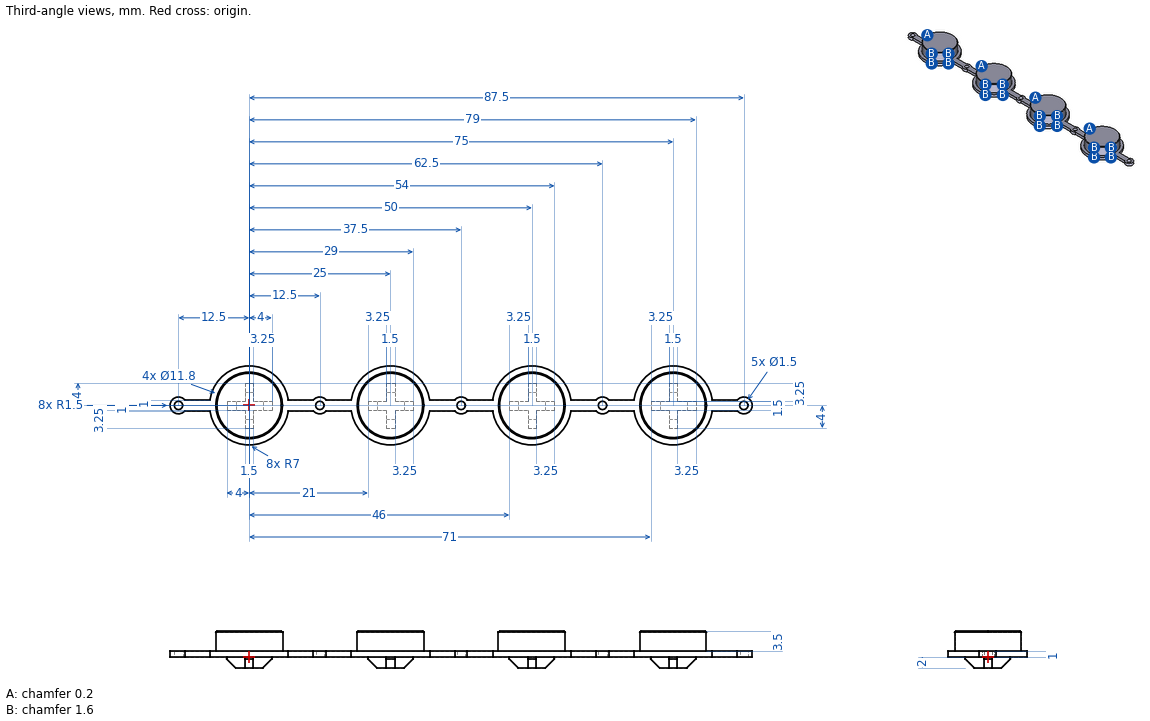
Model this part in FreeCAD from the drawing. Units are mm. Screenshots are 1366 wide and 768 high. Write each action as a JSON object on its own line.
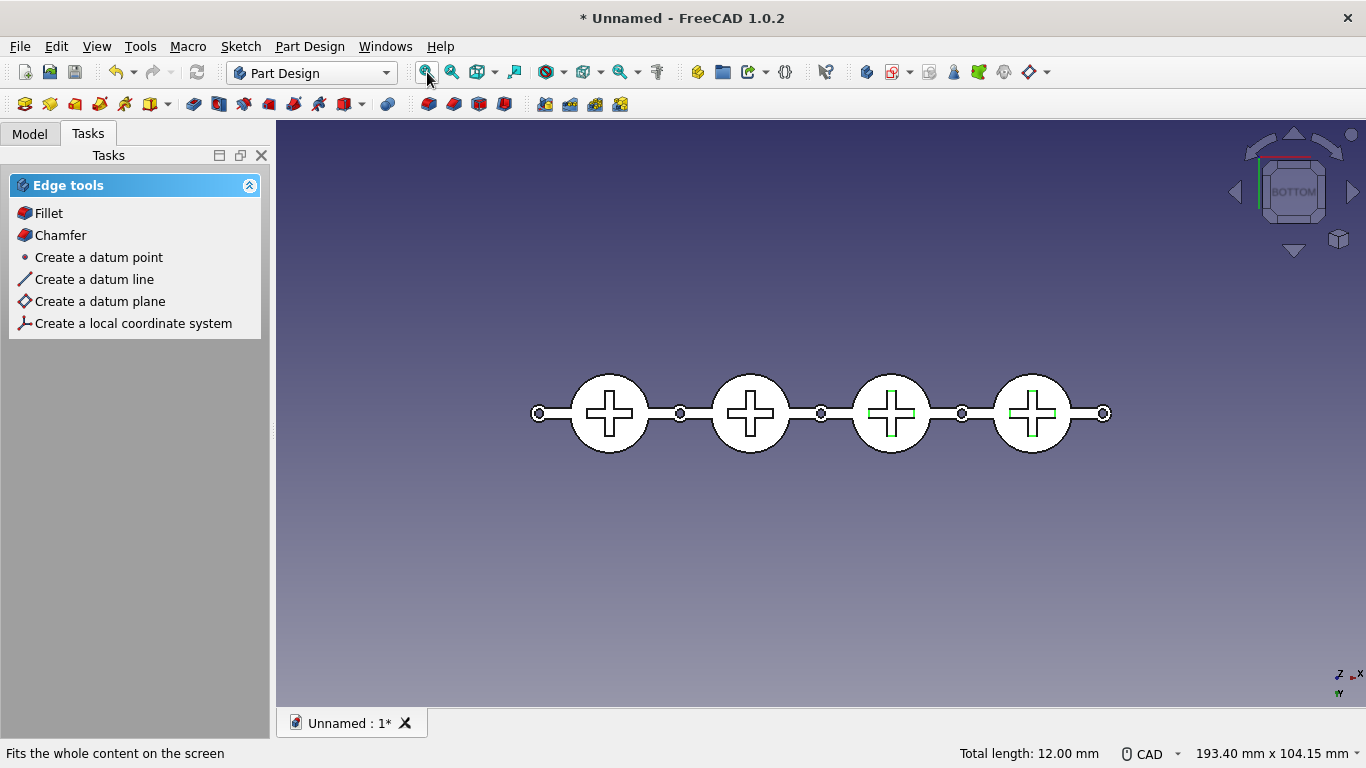
{"action": "key", "text": "4"}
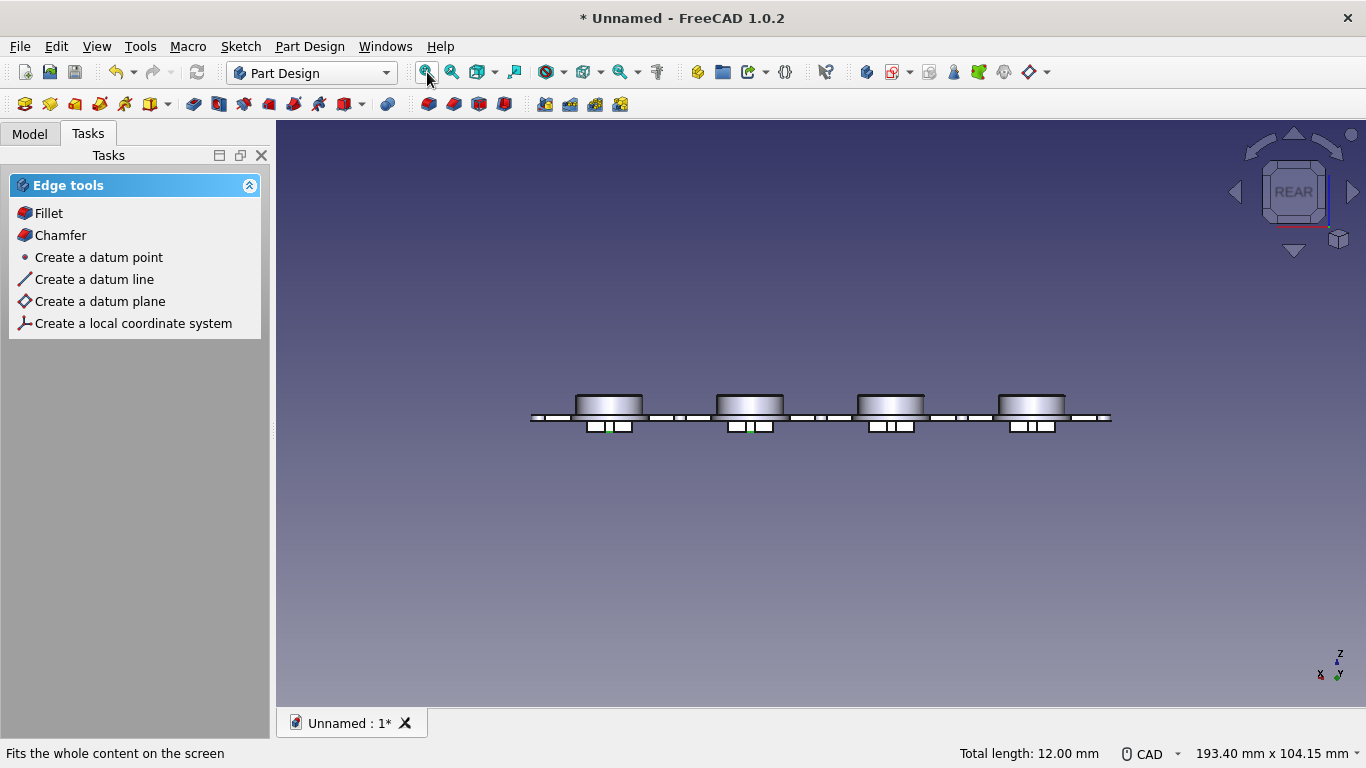
{"action": "scroll", "coordinate": [914, 431], "scroll_direction": "up", "scroll_amount": 8}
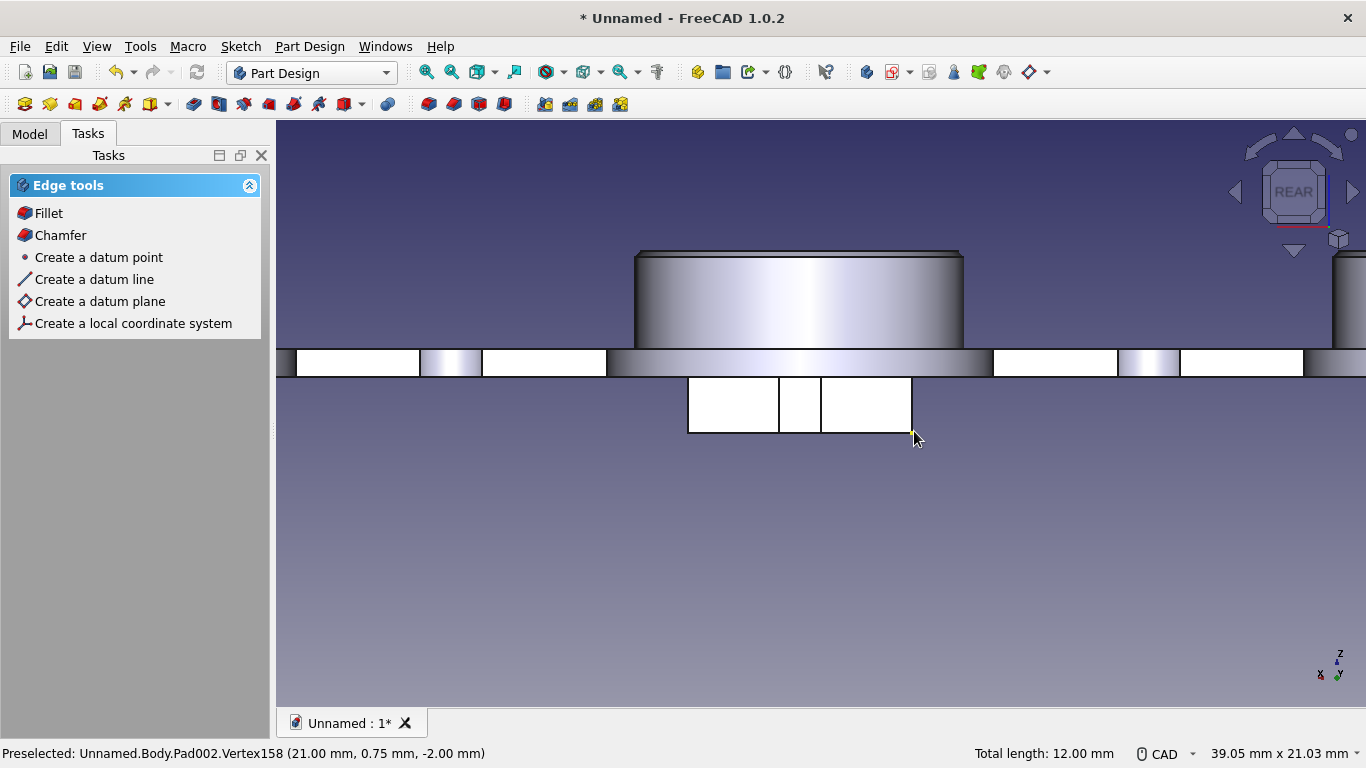
{"action": "left_click", "coordinate": [800, 432], "text": "ctrl"}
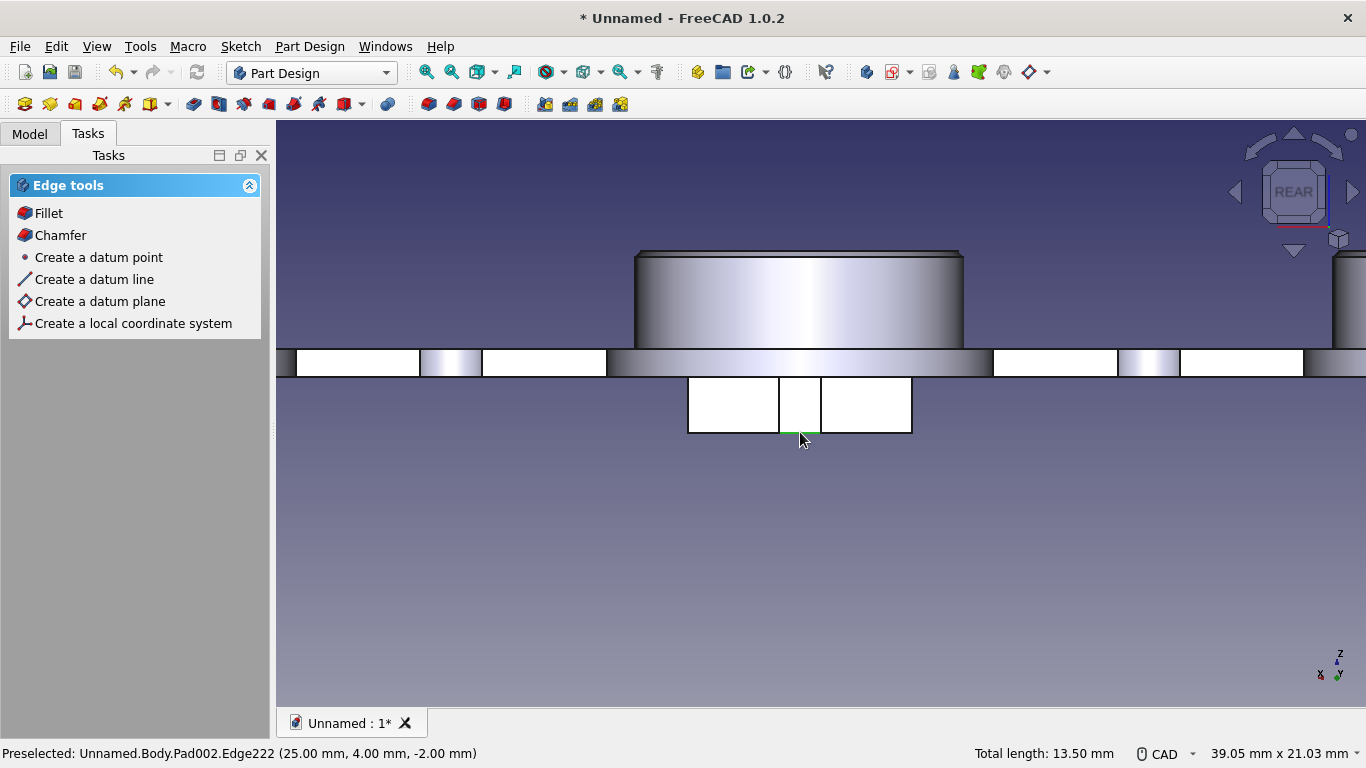
{"action": "key", "text": "v f"}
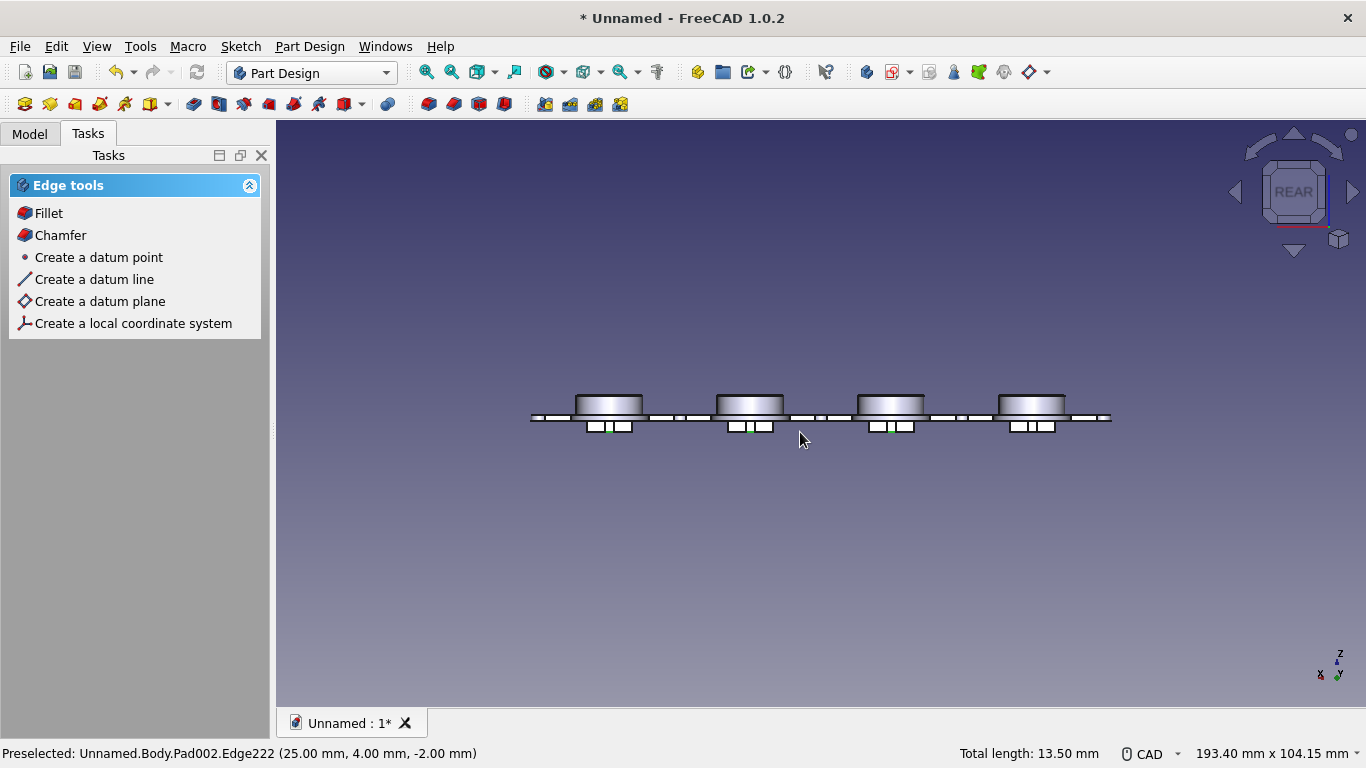
{"action": "key", "text": "6"}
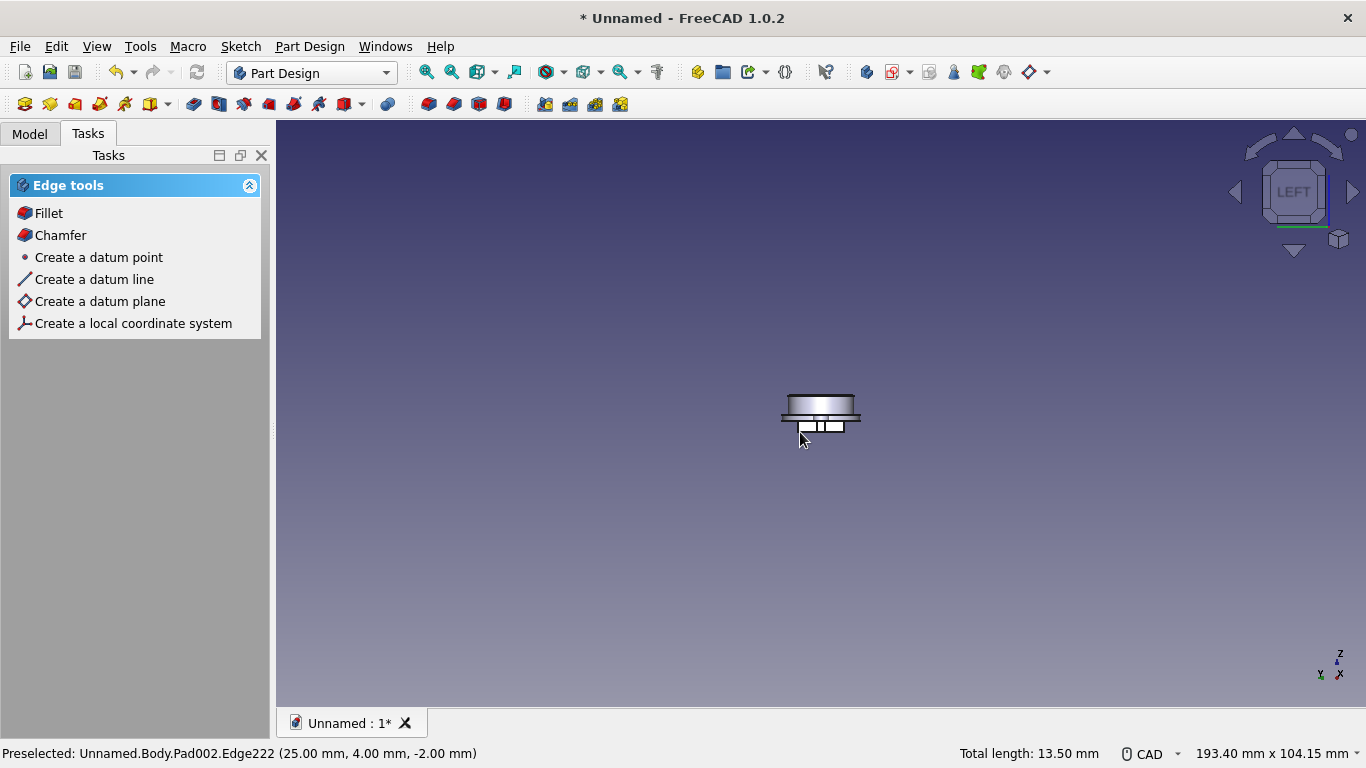
{"action": "key", "text": "v f"}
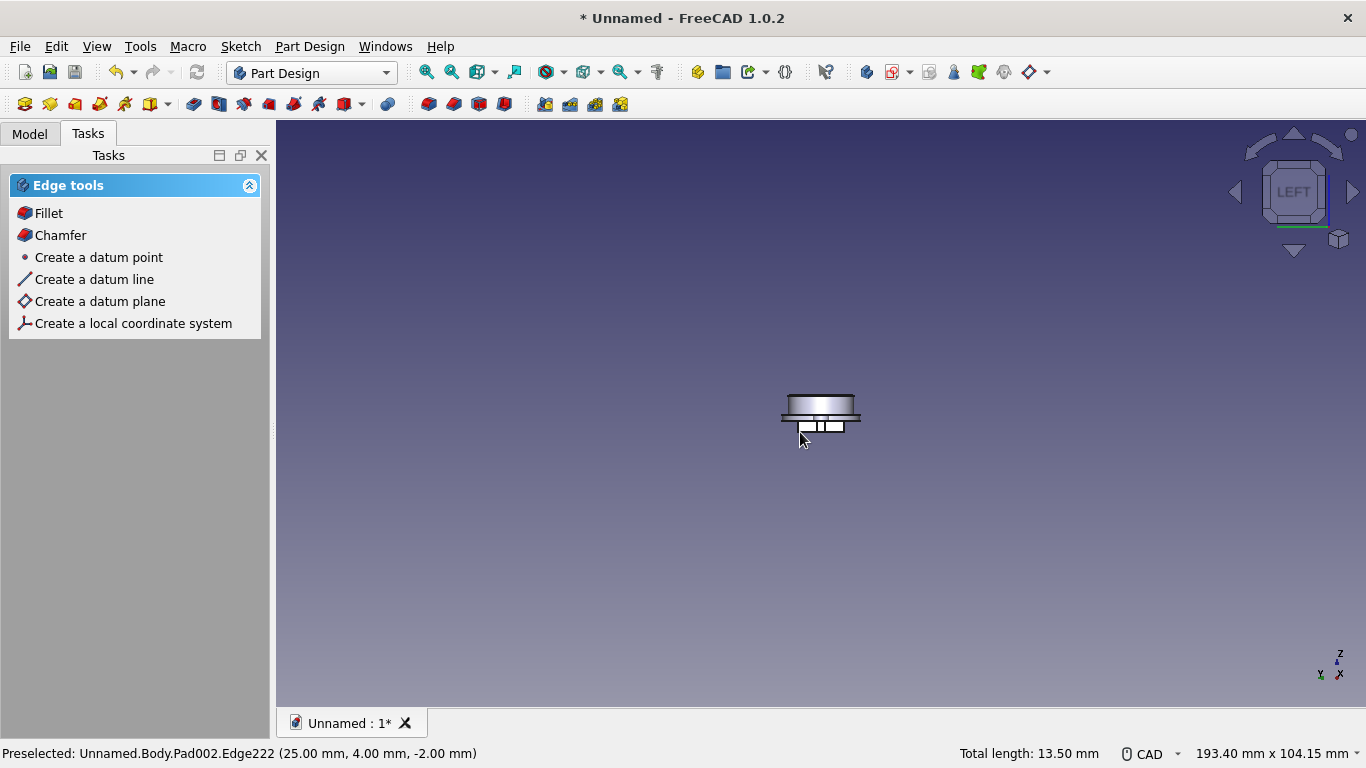
{"action": "scroll", "coordinate": [821, 431], "scroll_direction": "up", "scroll_amount": 8}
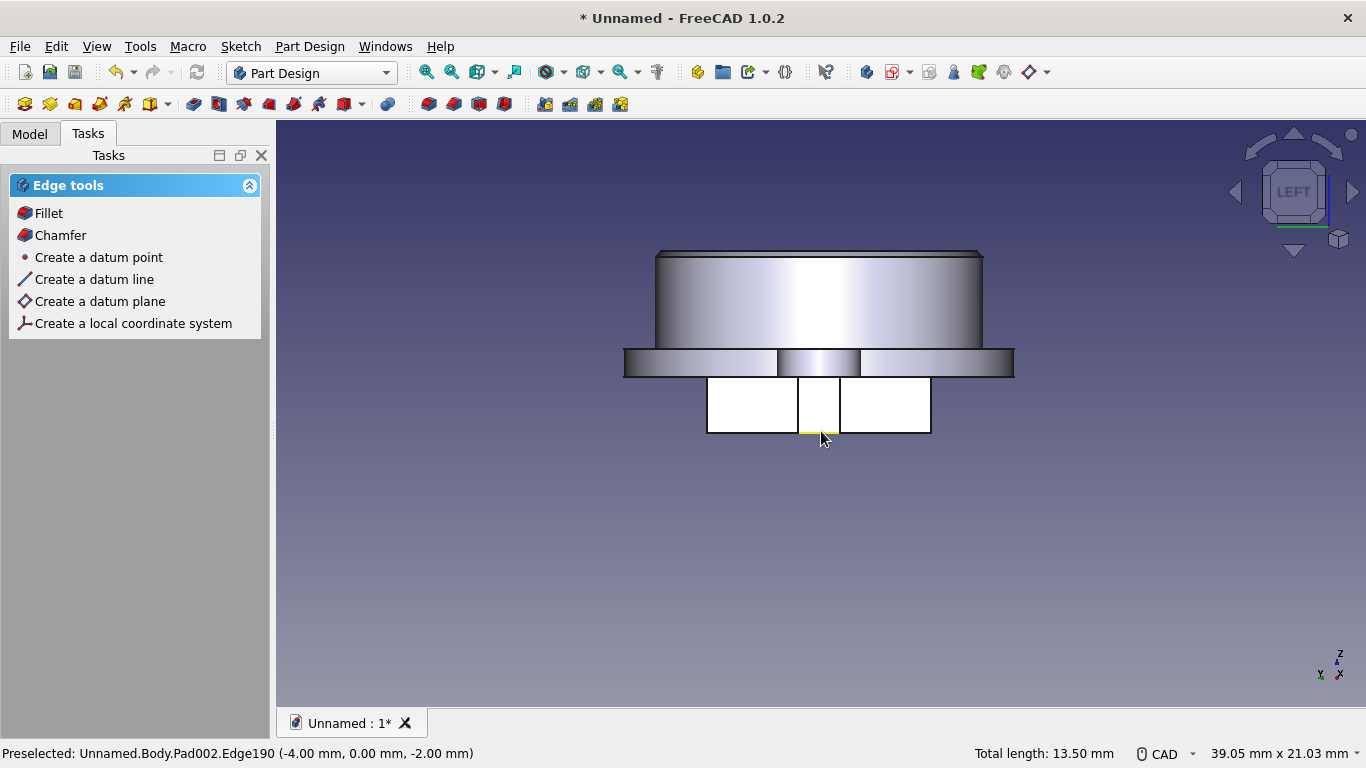
{"action": "left_click", "coordinate": [819, 432], "text": "ctrl"}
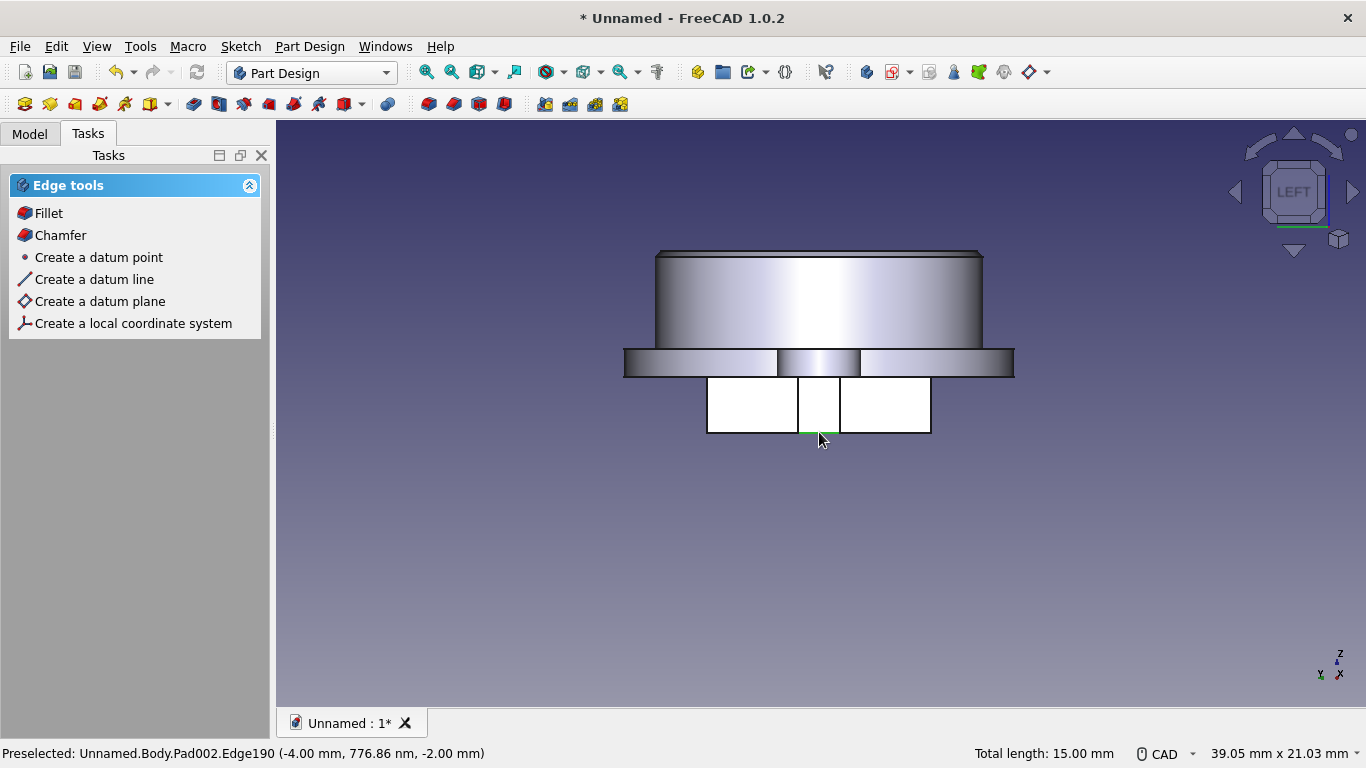
{"action": "key", "text": "v f"}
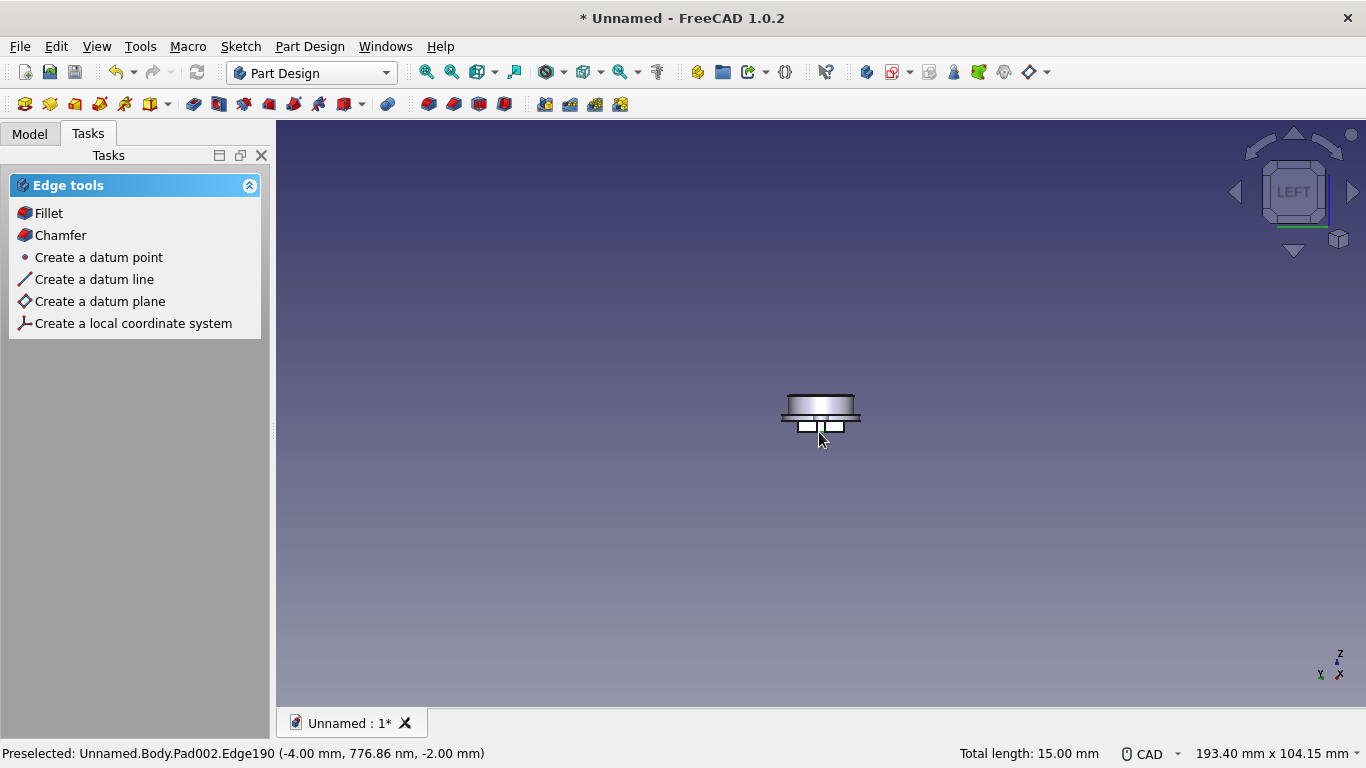
{"action": "key", "text": "v 3"}